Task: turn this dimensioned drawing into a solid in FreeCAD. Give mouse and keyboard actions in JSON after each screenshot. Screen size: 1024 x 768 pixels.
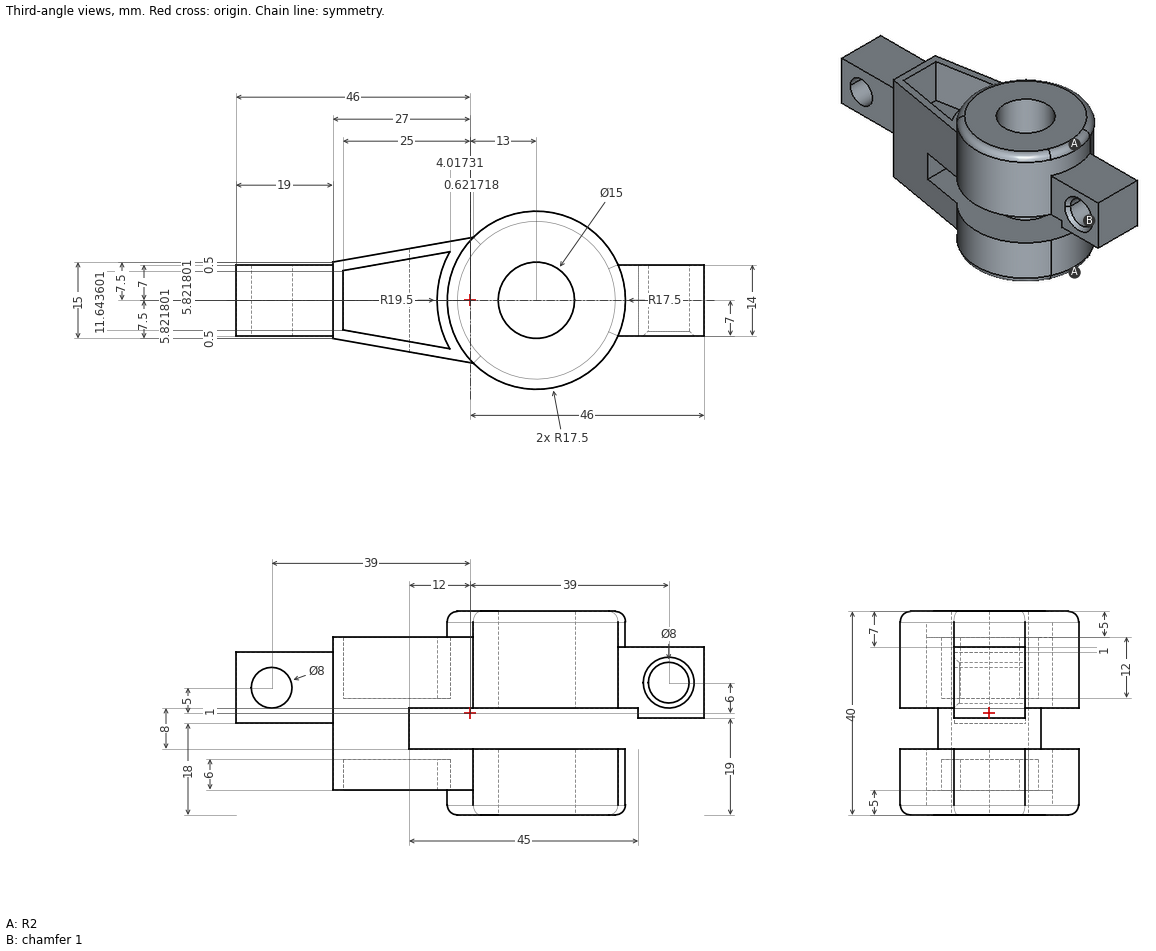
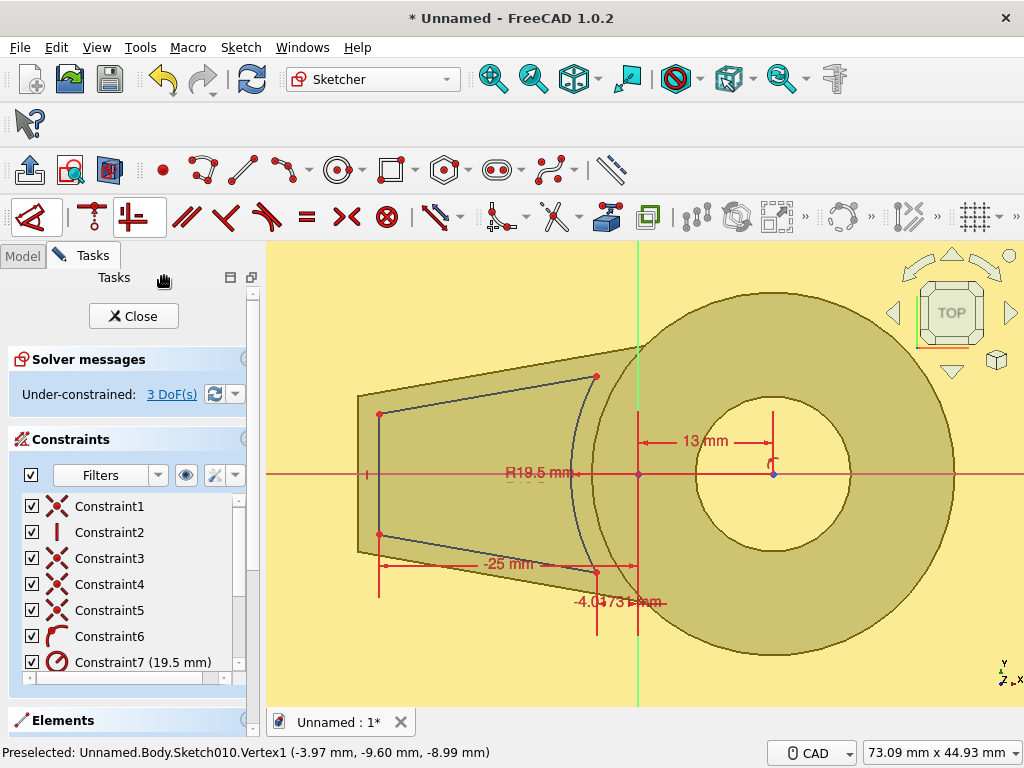
{"action": "left_click", "coordinate": [596, 376]}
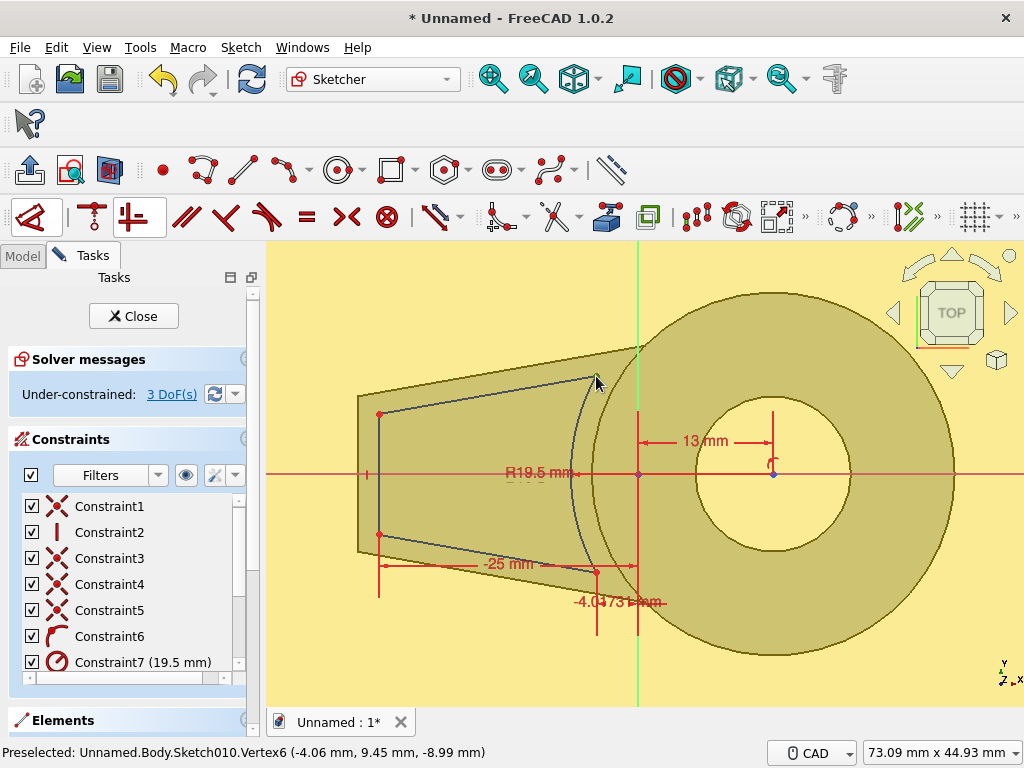
{"action": "left_click", "coordinate": [56, 218]}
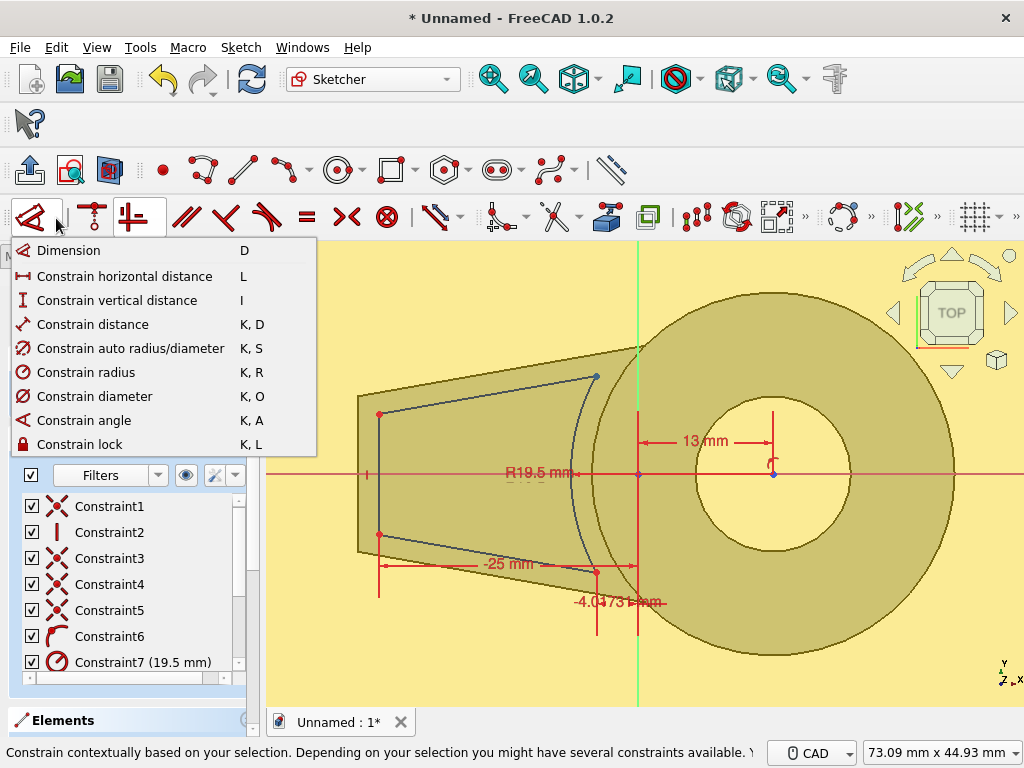
{"action": "left_click", "coordinate": [164, 276]}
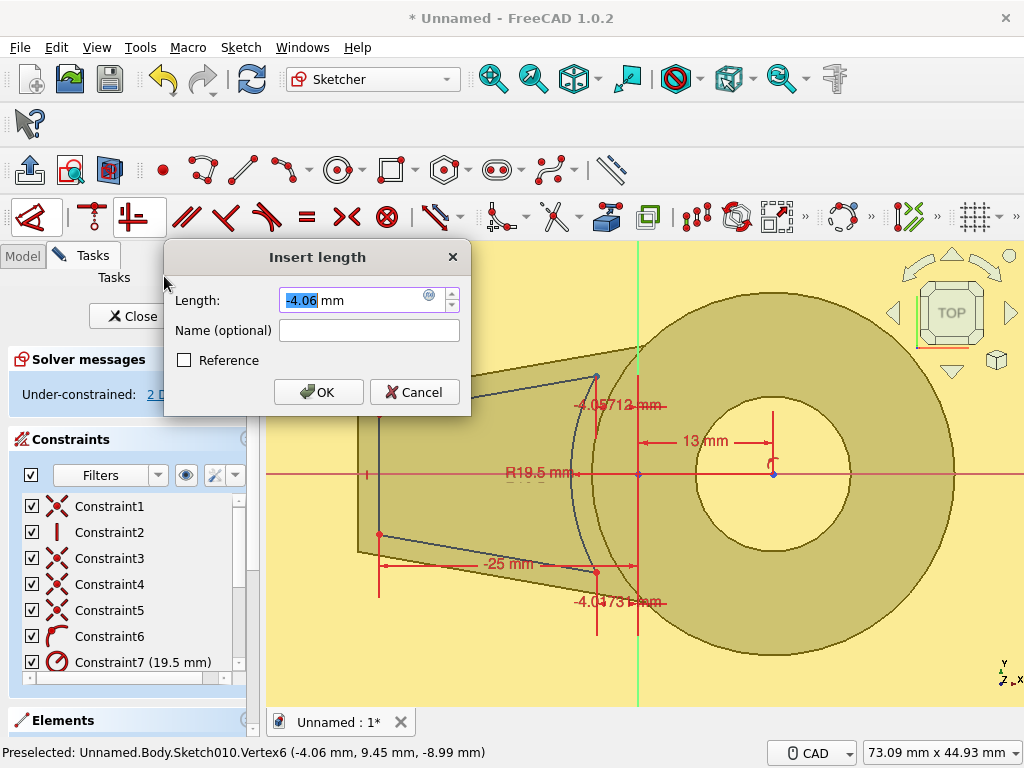
{"action": "type", "text": "-4.01731"}
{"action": "key", "text": "Return"}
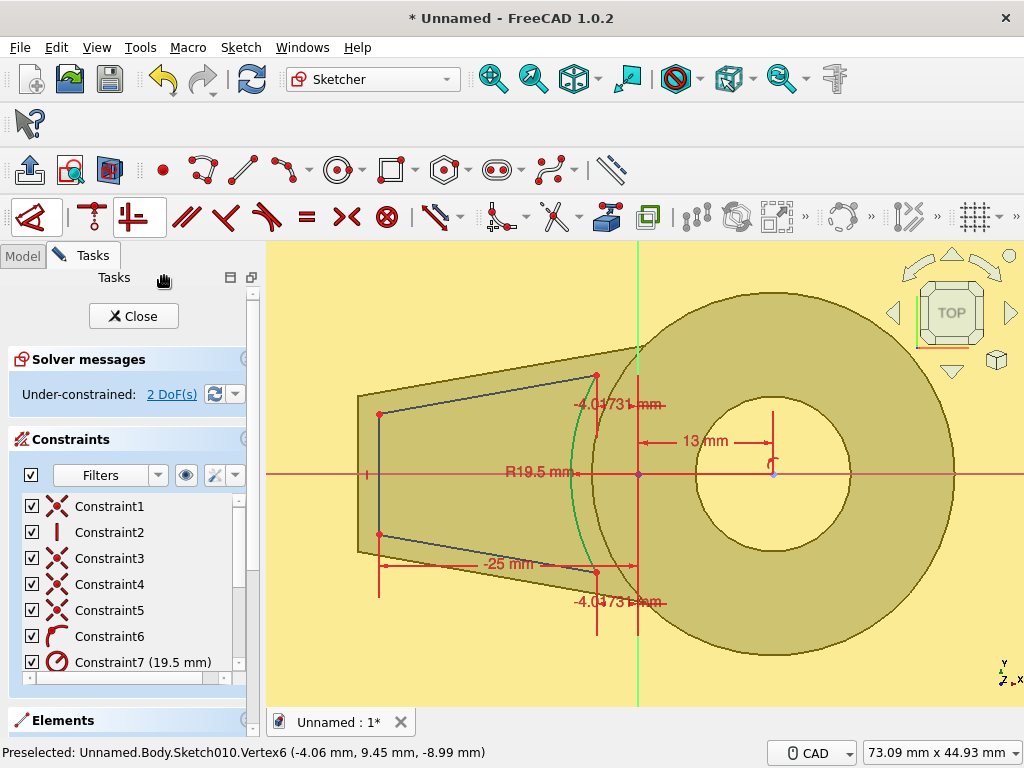
{"action": "left_click", "coordinate": [379, 499]}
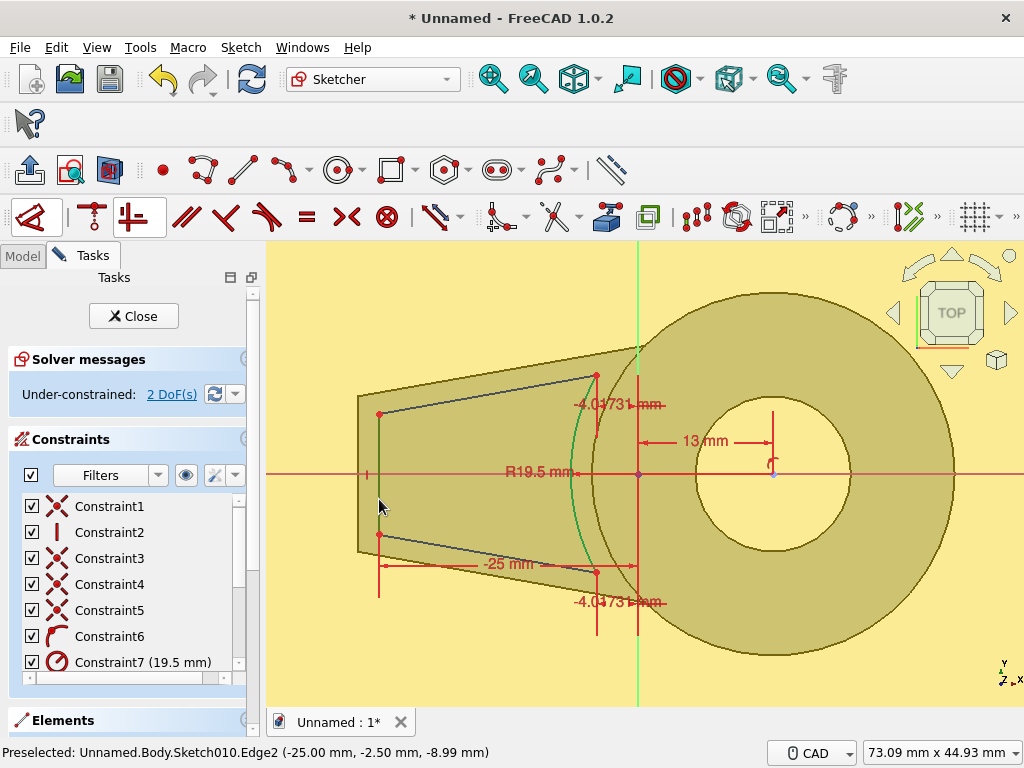
{"action": "left_click", "coordinate": [56, 218]}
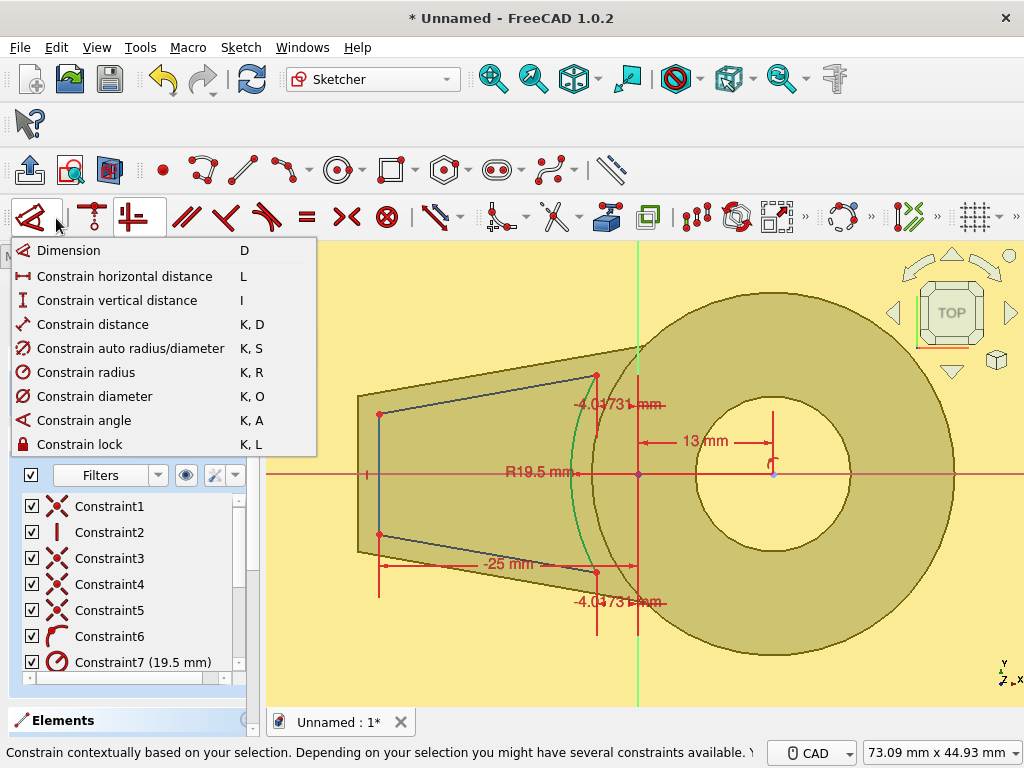
{"action": "left_click", "coordinate": [164, 300]}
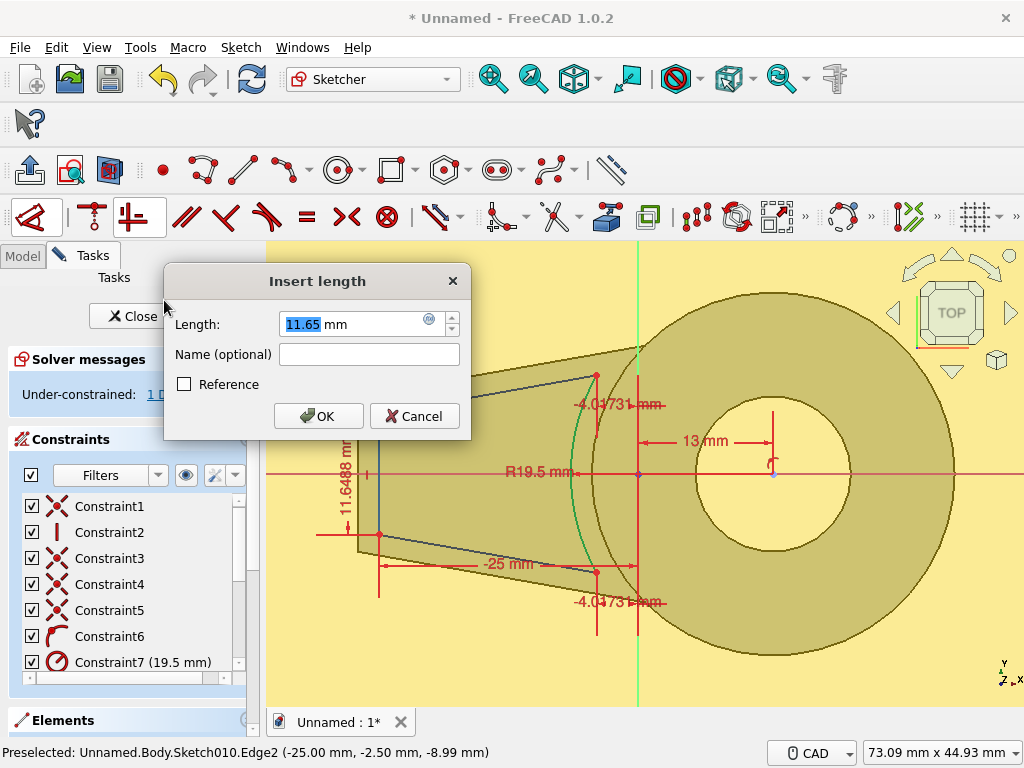
{"action": "type", "text": "11.643601"}
{"action": "key", "text": "Return"}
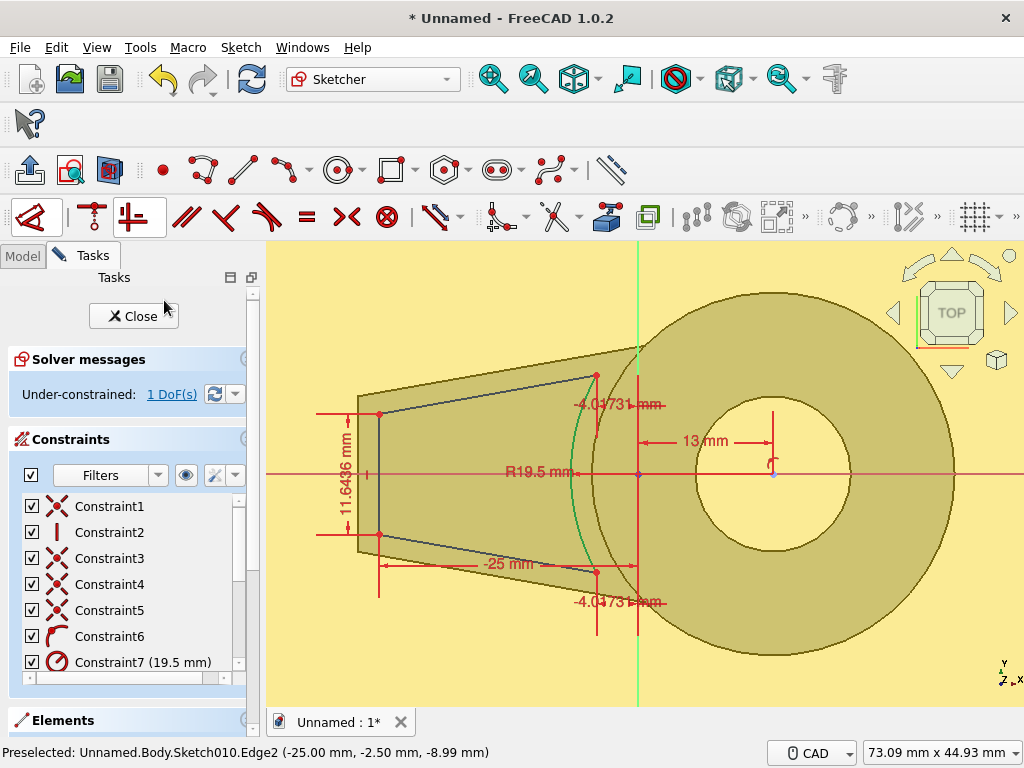
{"action": "left_click", "coordinate": [379, 535]}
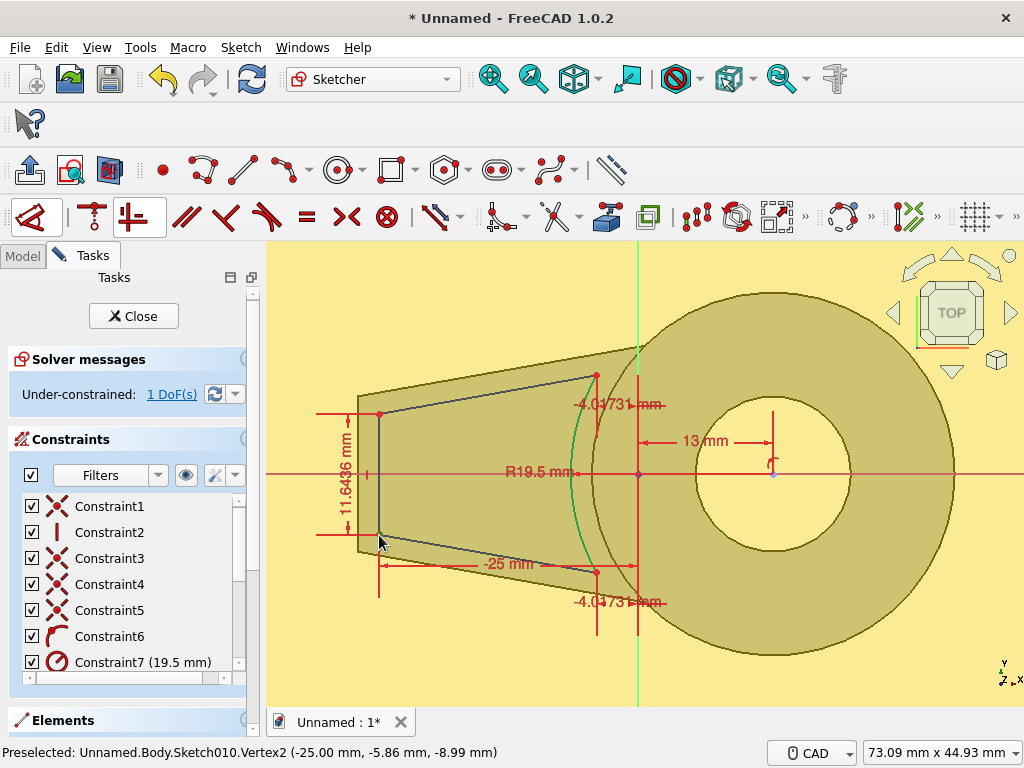
{"action": "left_click", "coordinate": [56, 218]}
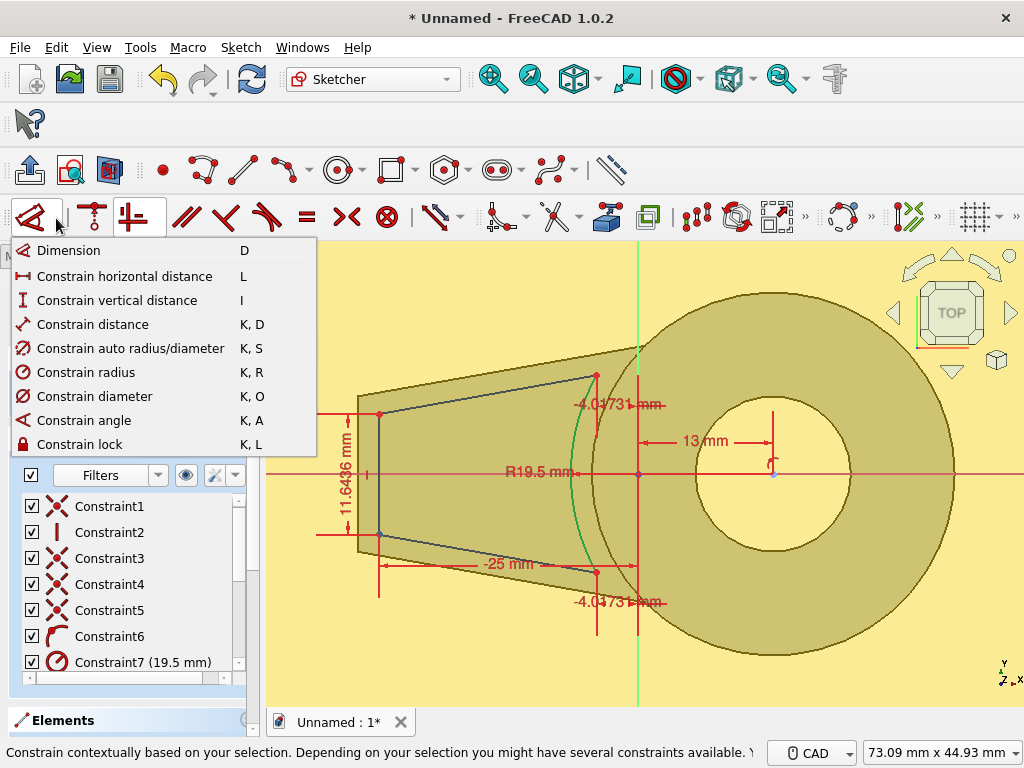
{"action": "left_click", "coordinate": [164, 300]}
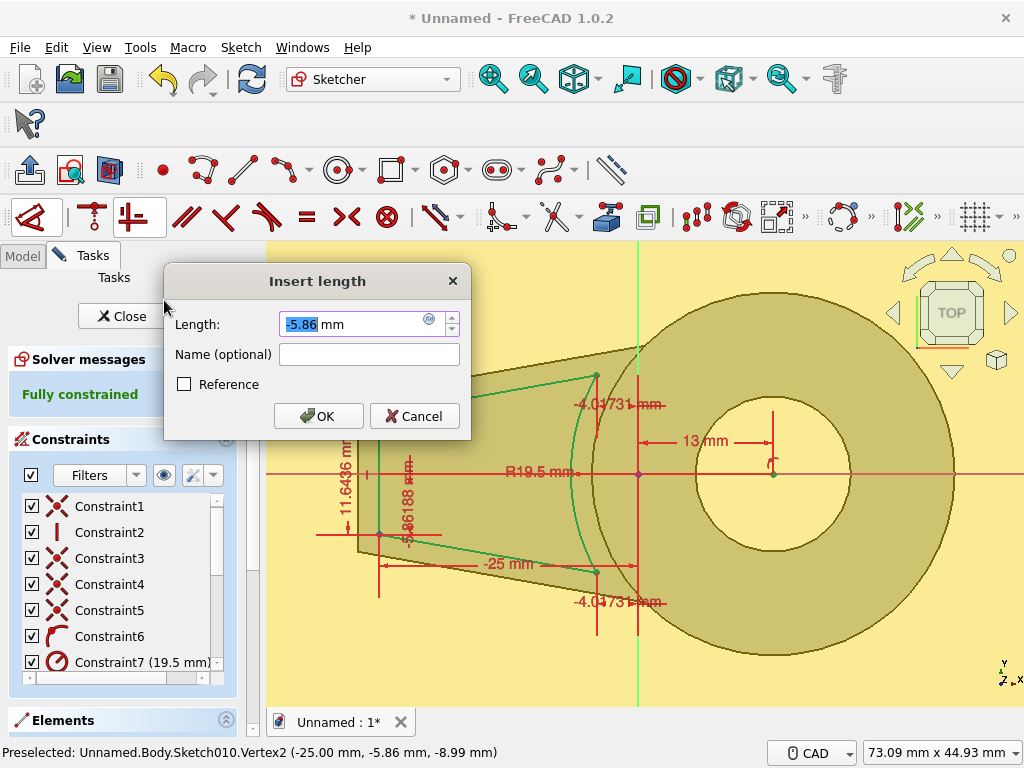
{"action": "type", "text": "-5.821801"}
{"action": "key", "text": "Return"}